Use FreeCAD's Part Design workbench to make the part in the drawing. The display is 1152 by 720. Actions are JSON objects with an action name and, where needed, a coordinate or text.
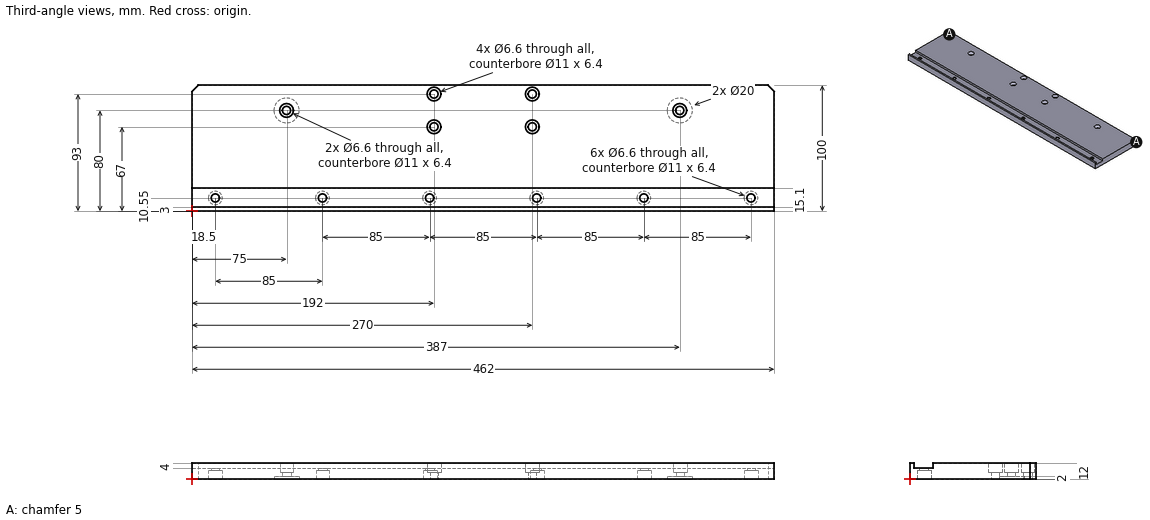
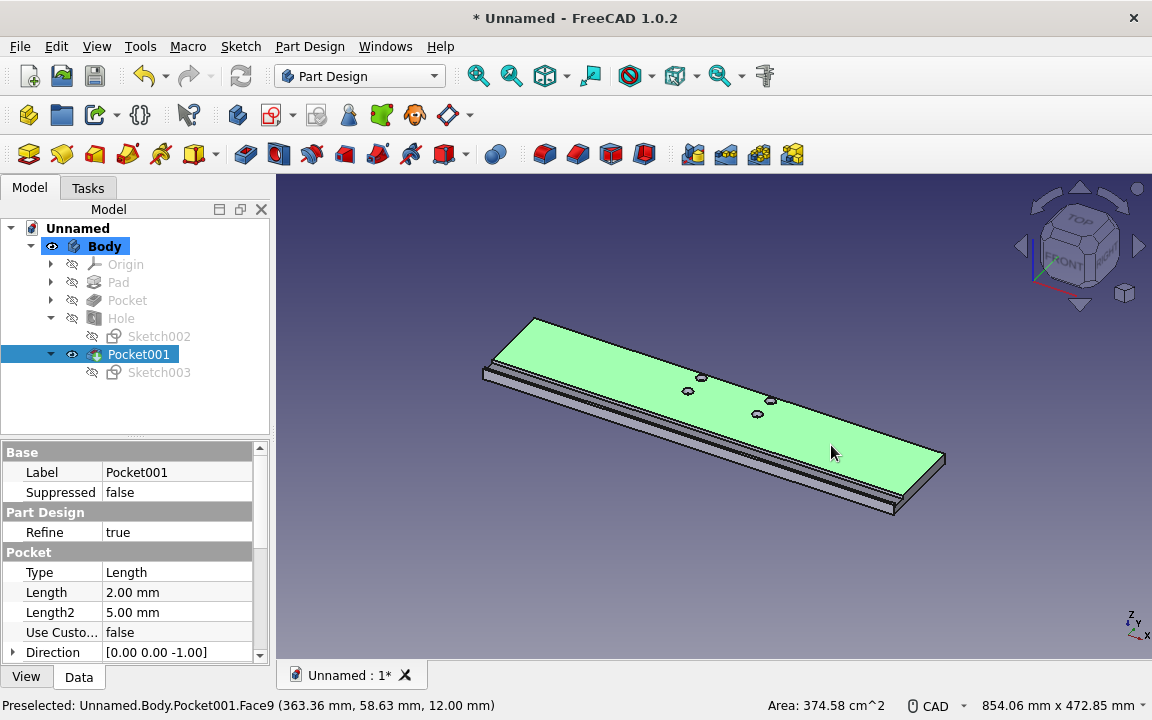
{"action": "left_click", "coordinate": [270, 116]}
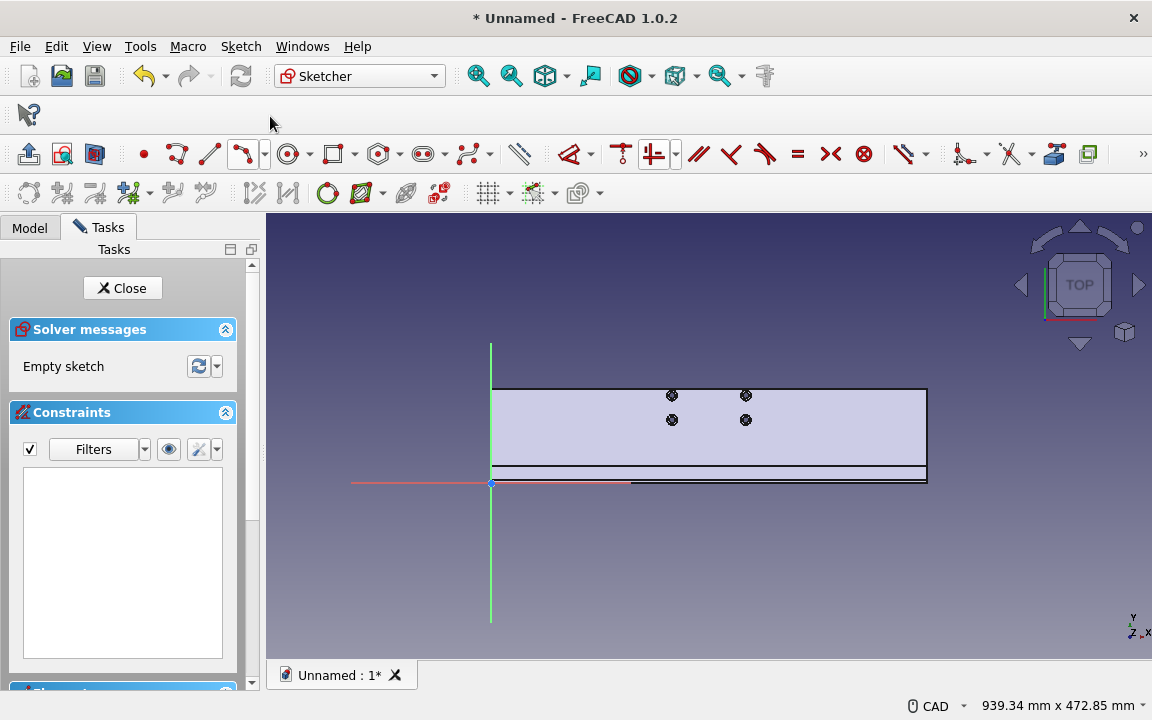
{"action": "key", "text": "g c"}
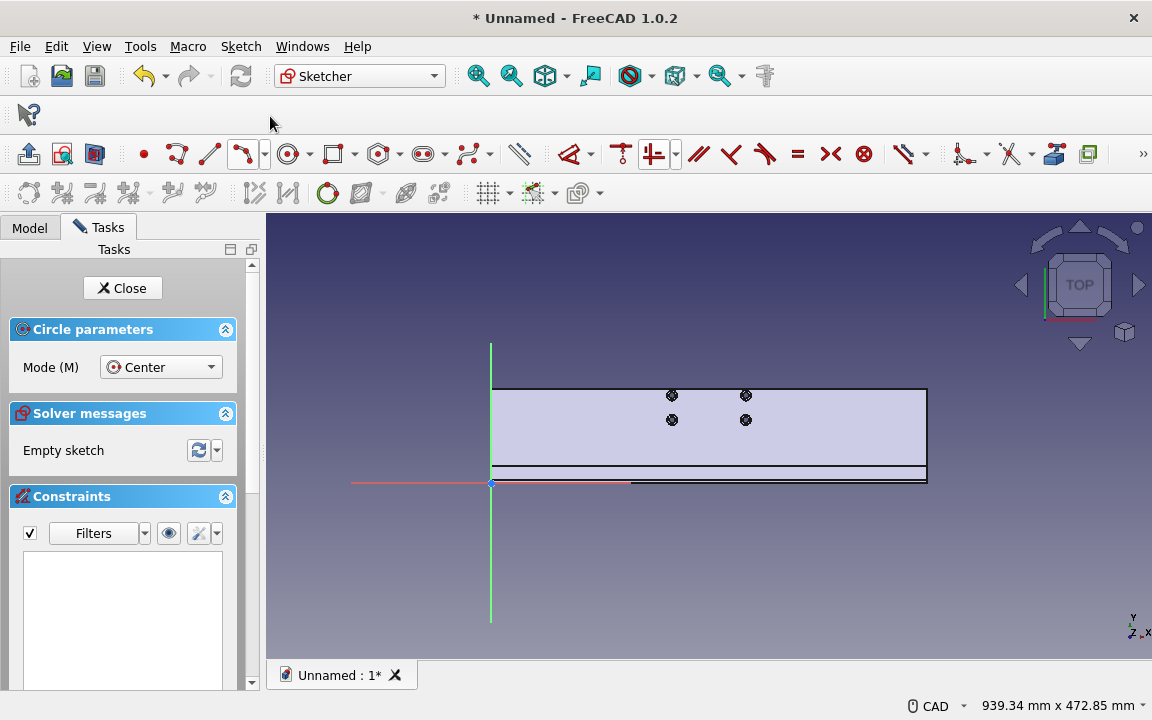
{"action": "scroll", "coordinate": [562, 408], "scroll_direction": "up", "scroll_amount": 10}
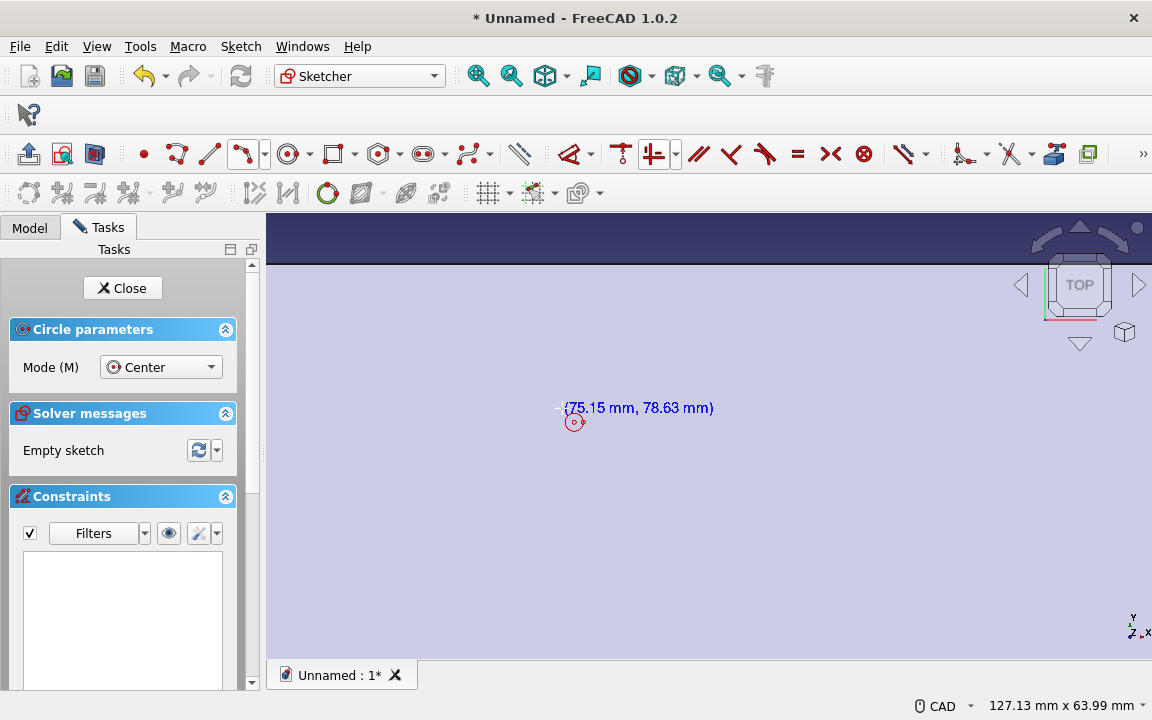
{"action": "scroll", "coordinate": [491, 390], "scroll_direction": "down", "scroll_amount": 9}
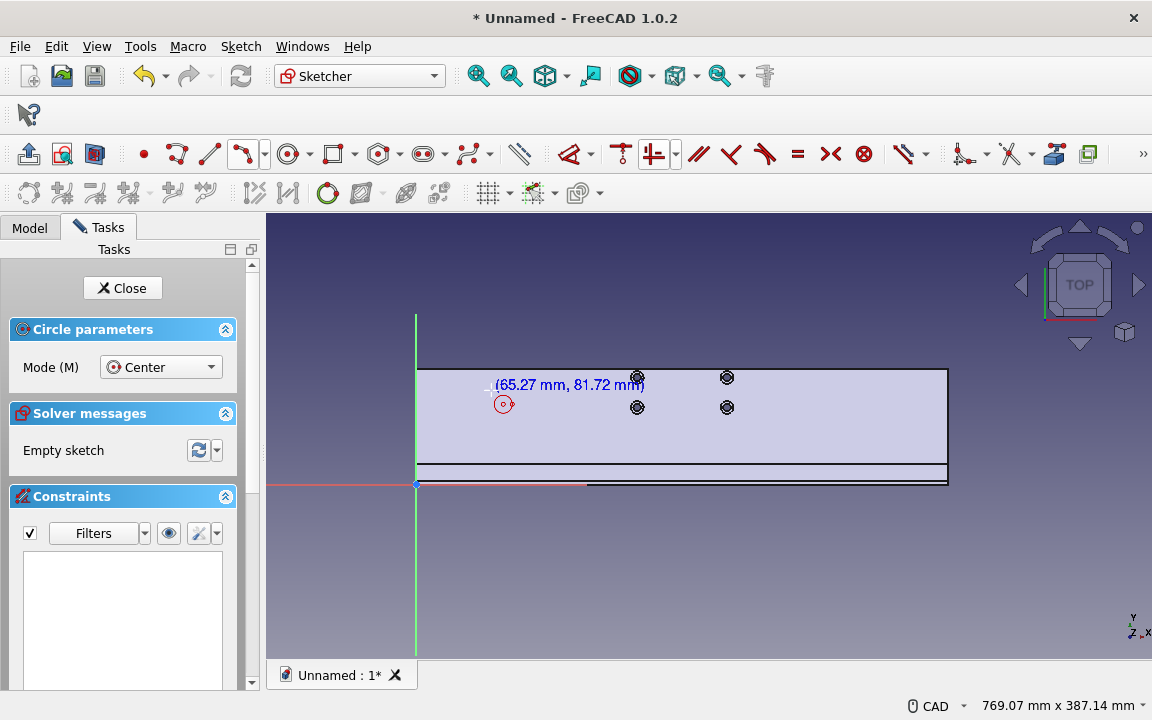
{"action": "left_click", "coordinate": [502, 392]}
{"action": "mouse_move", "coordinate": [505, 390]}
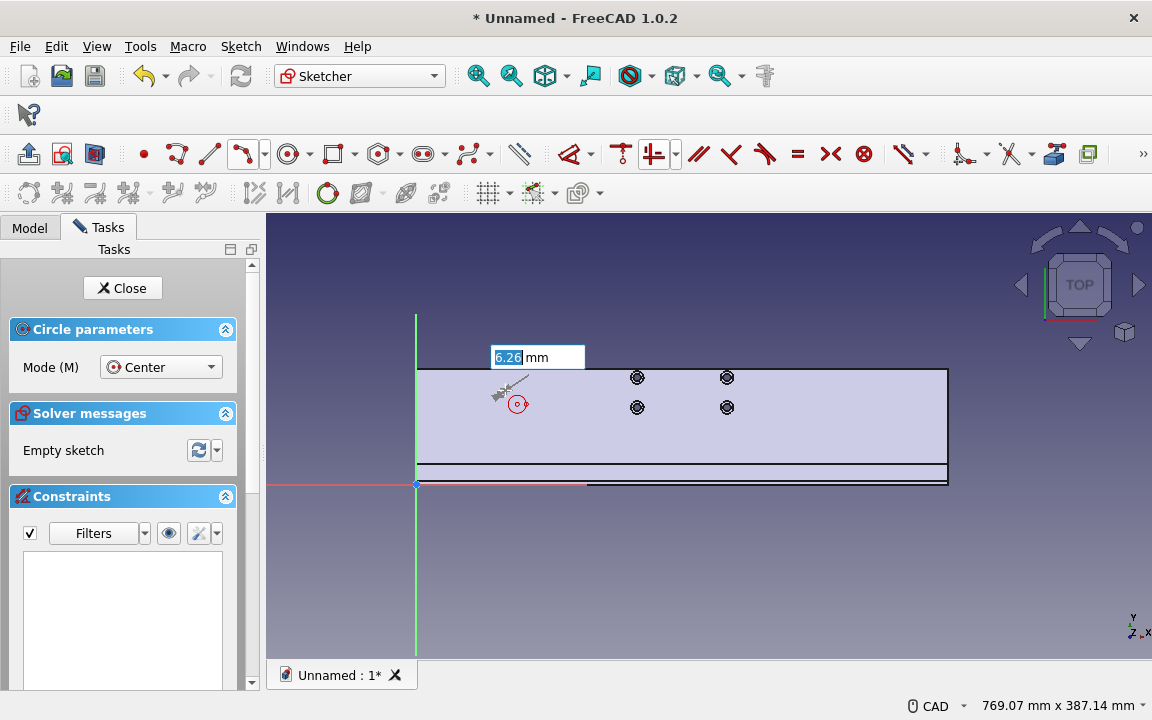
{"action": "type", "text": "6.6"}
{"action": "key", "text": "Return"}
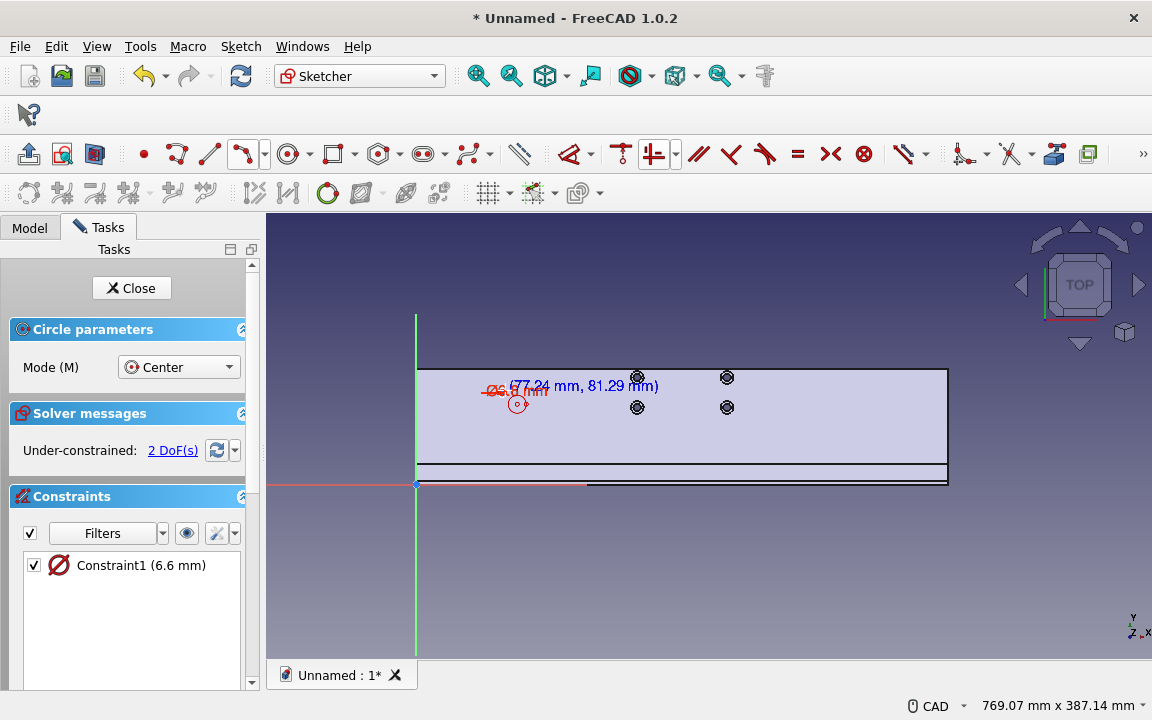
{"action": "scroll", "coordinate": [862, 392], "scroll_direction": "up", "scroll_amount": 9}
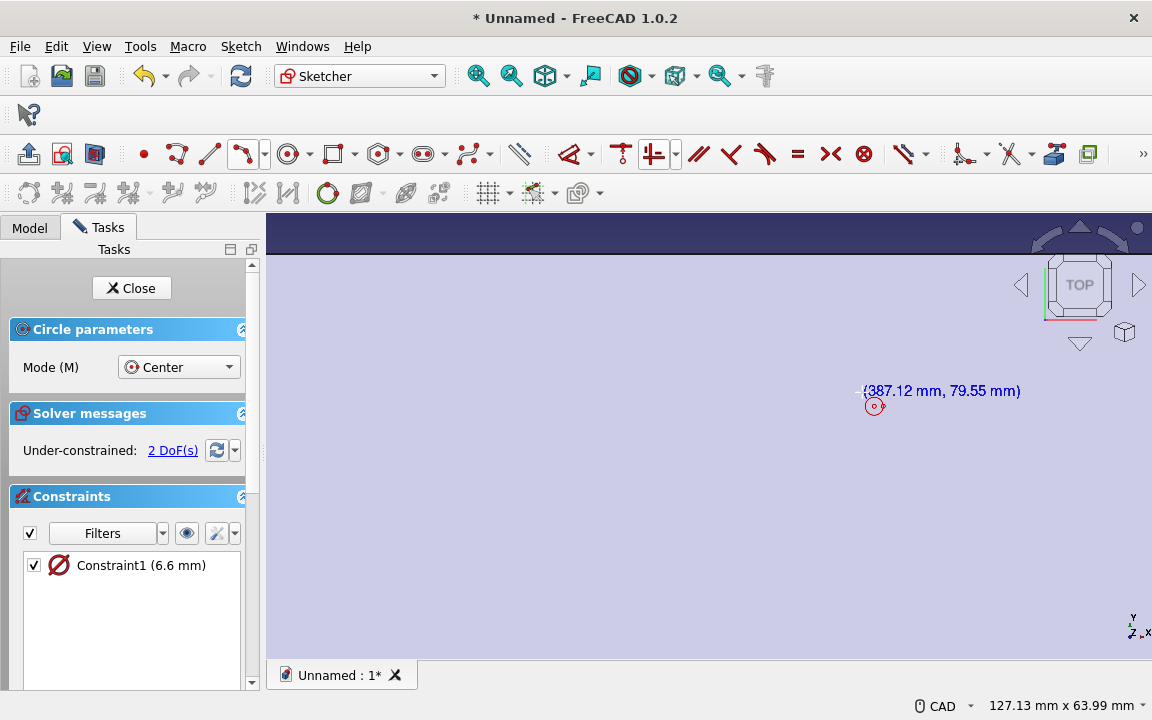
{"action": "scroll", "coordinate": [862, 392], "scroll_direction": "down", "scroll_amount": 9}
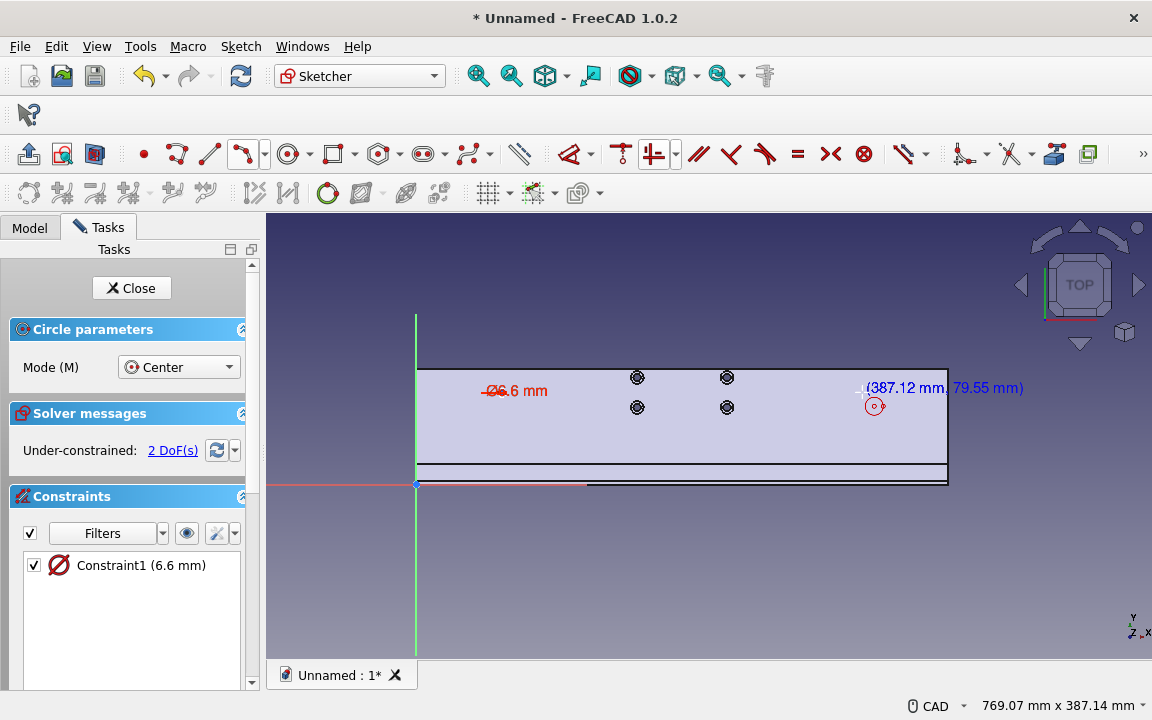
{"action": "left_click", "coordinate": [862, 392]}
{"action": "mouse_move", "coordinate": [865, 390]}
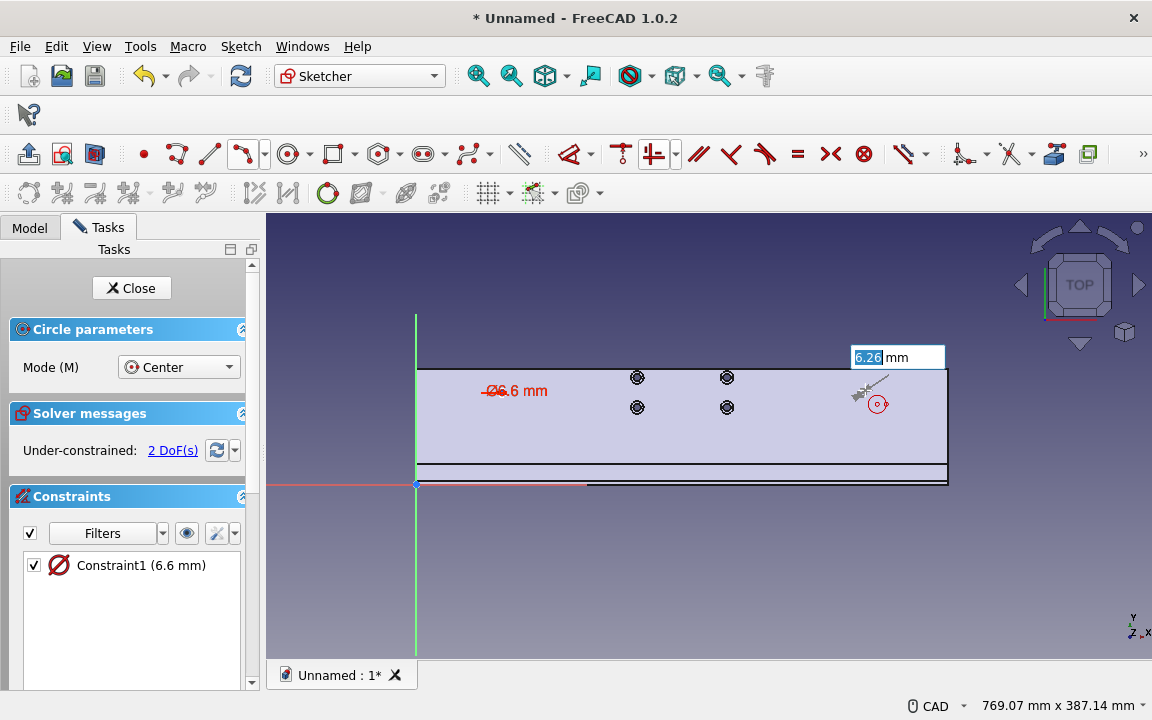
{"action": "type", "text": "6.6"}
{"action": "key", "text": "Return"}
{"action": "key", "text": "Escape"}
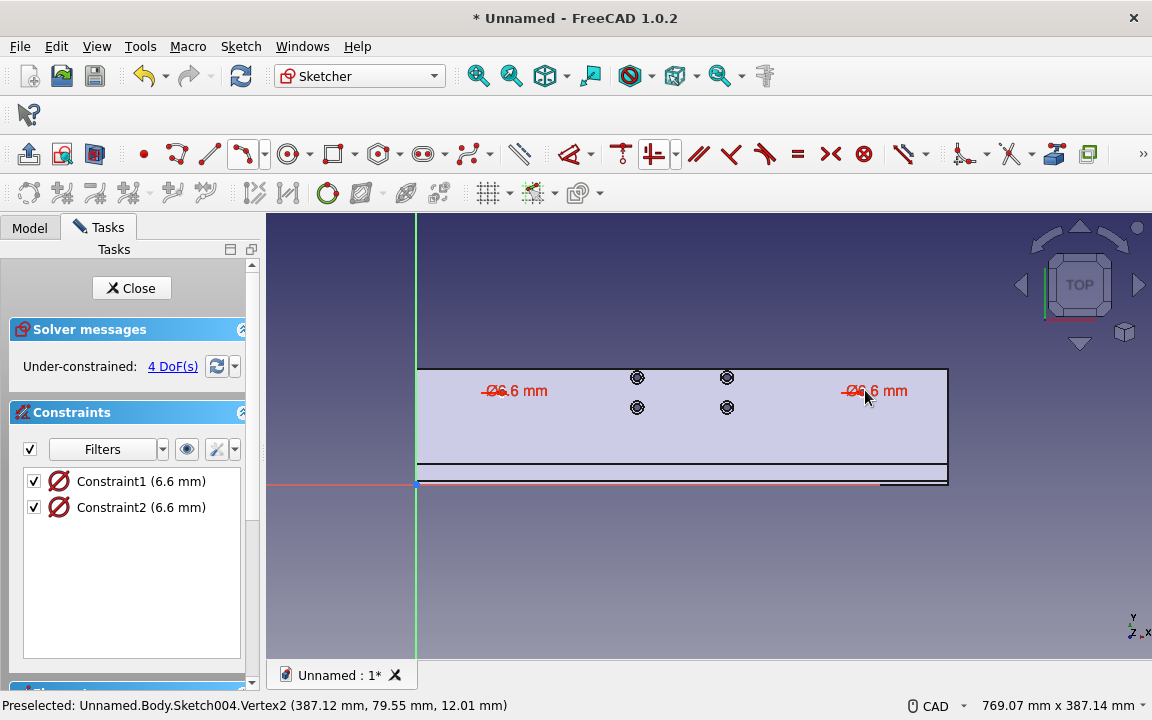
{"action": "left_click", "coordinate": [502, 393]}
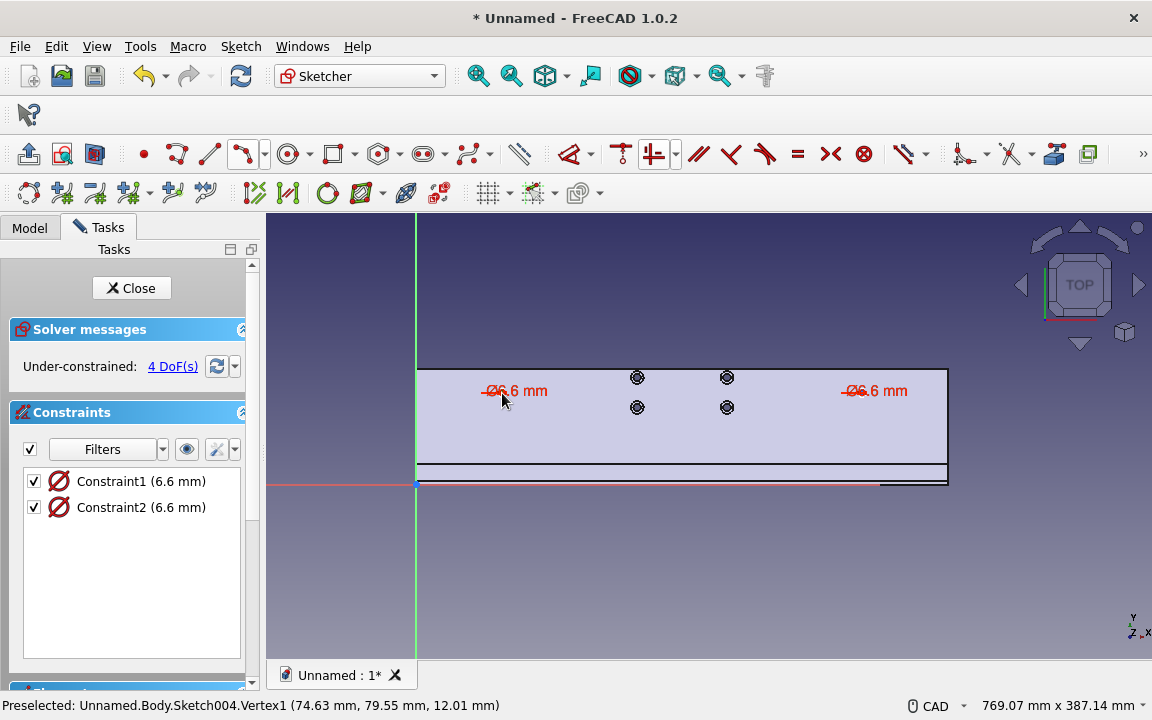
{"action": "left_click", "coordinate": [862, 393]}